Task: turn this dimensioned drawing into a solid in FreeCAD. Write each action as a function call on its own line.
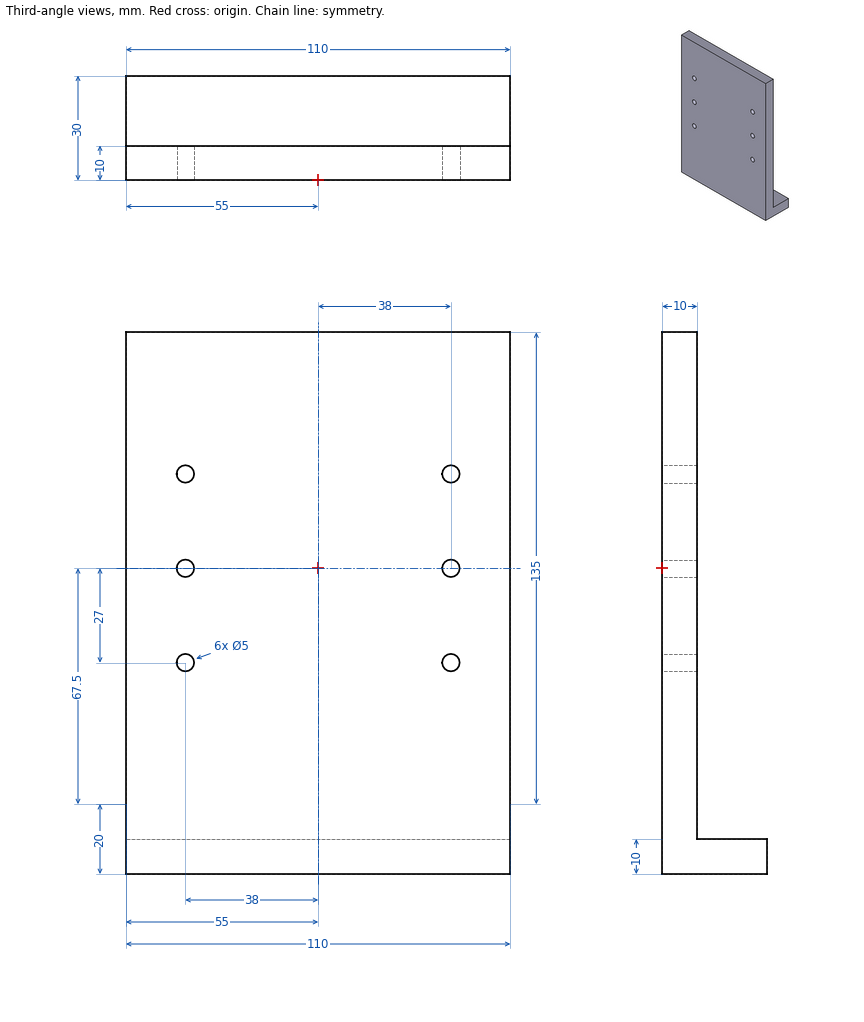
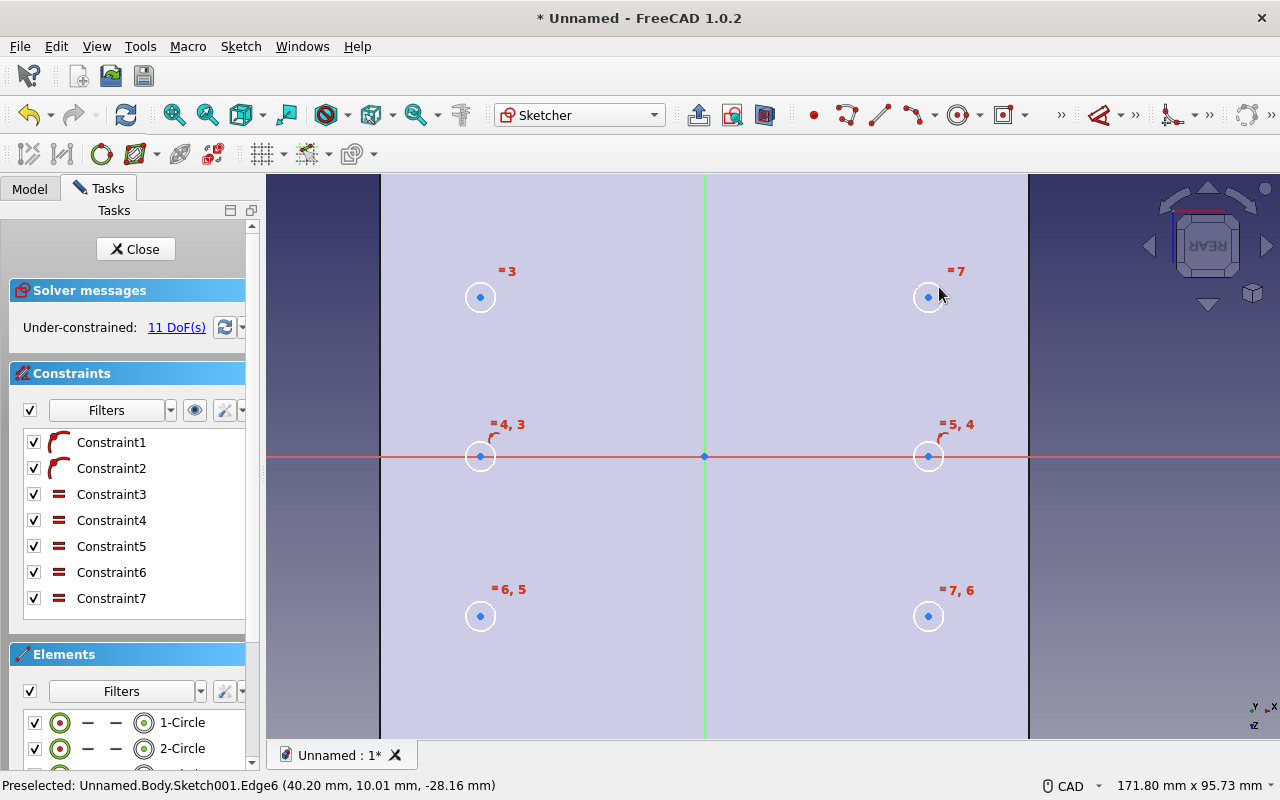
click(481, 298)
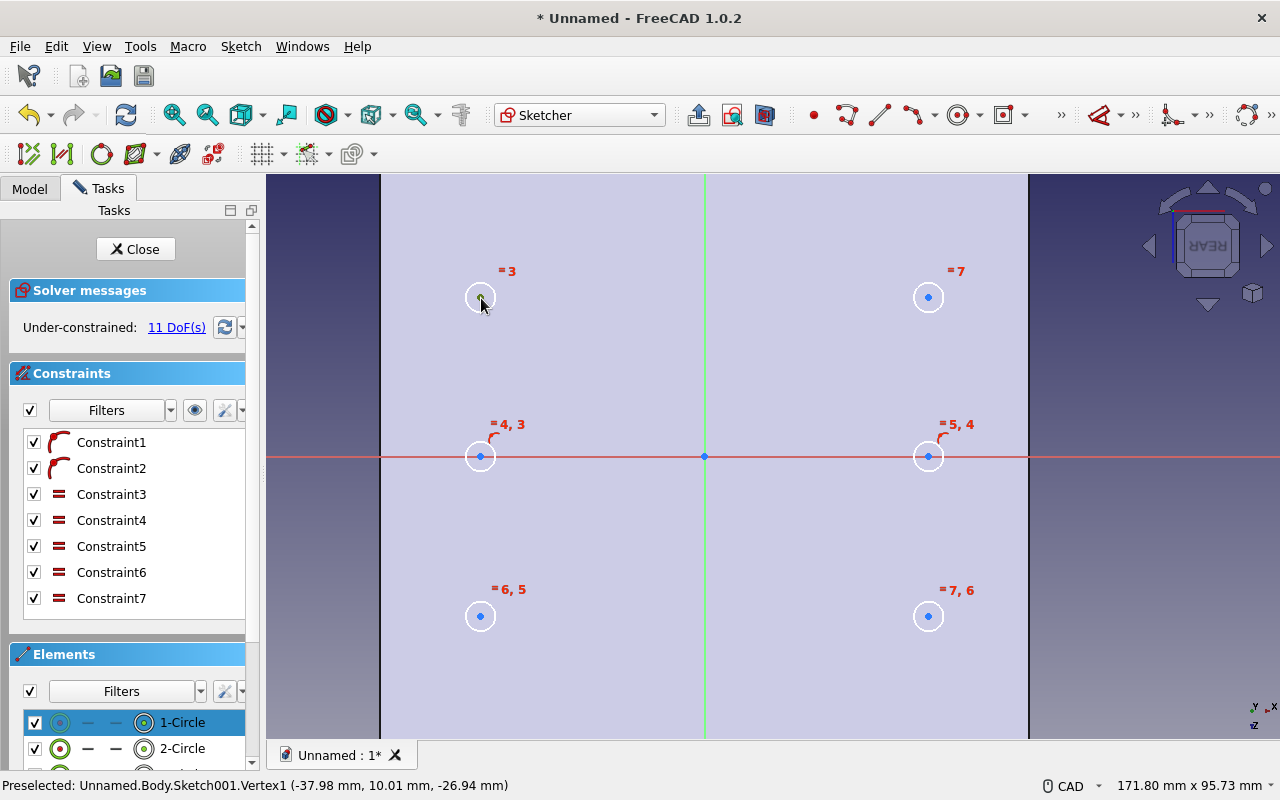
click(481, 616)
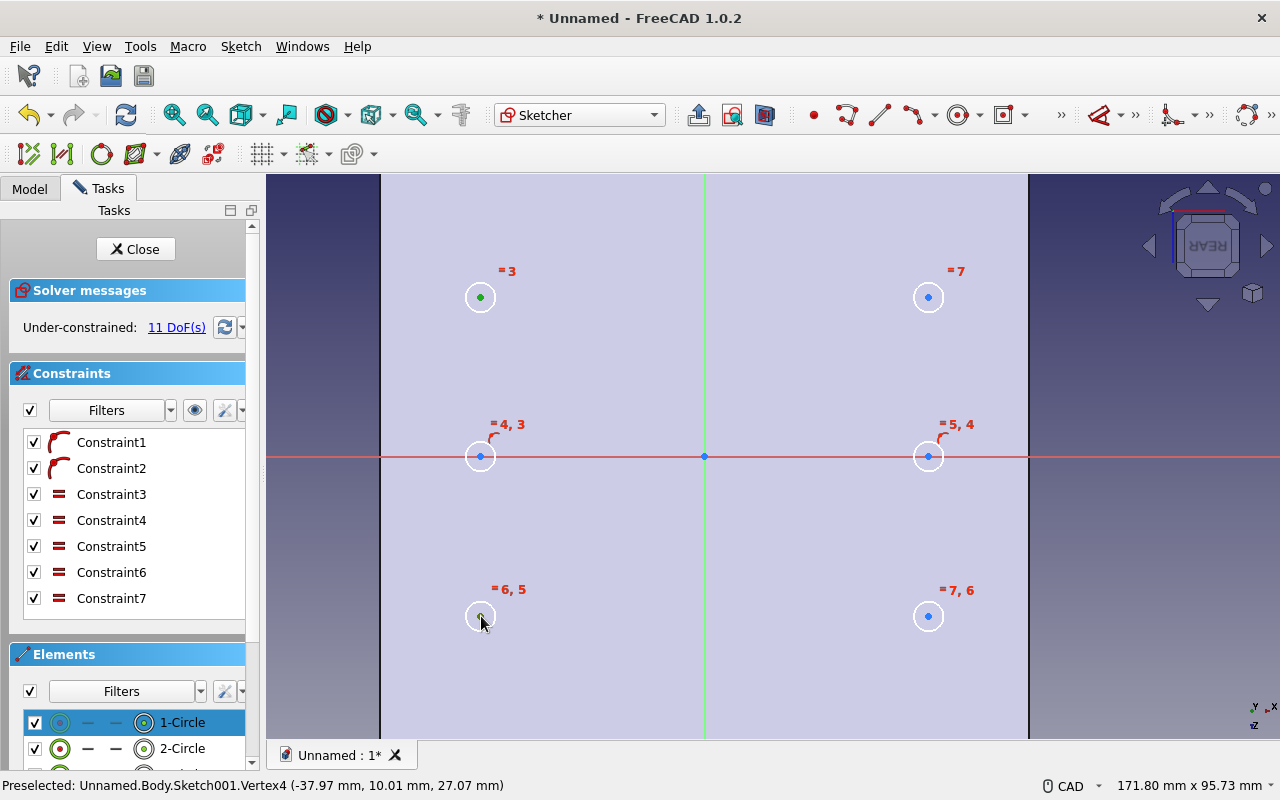
click(353, 457)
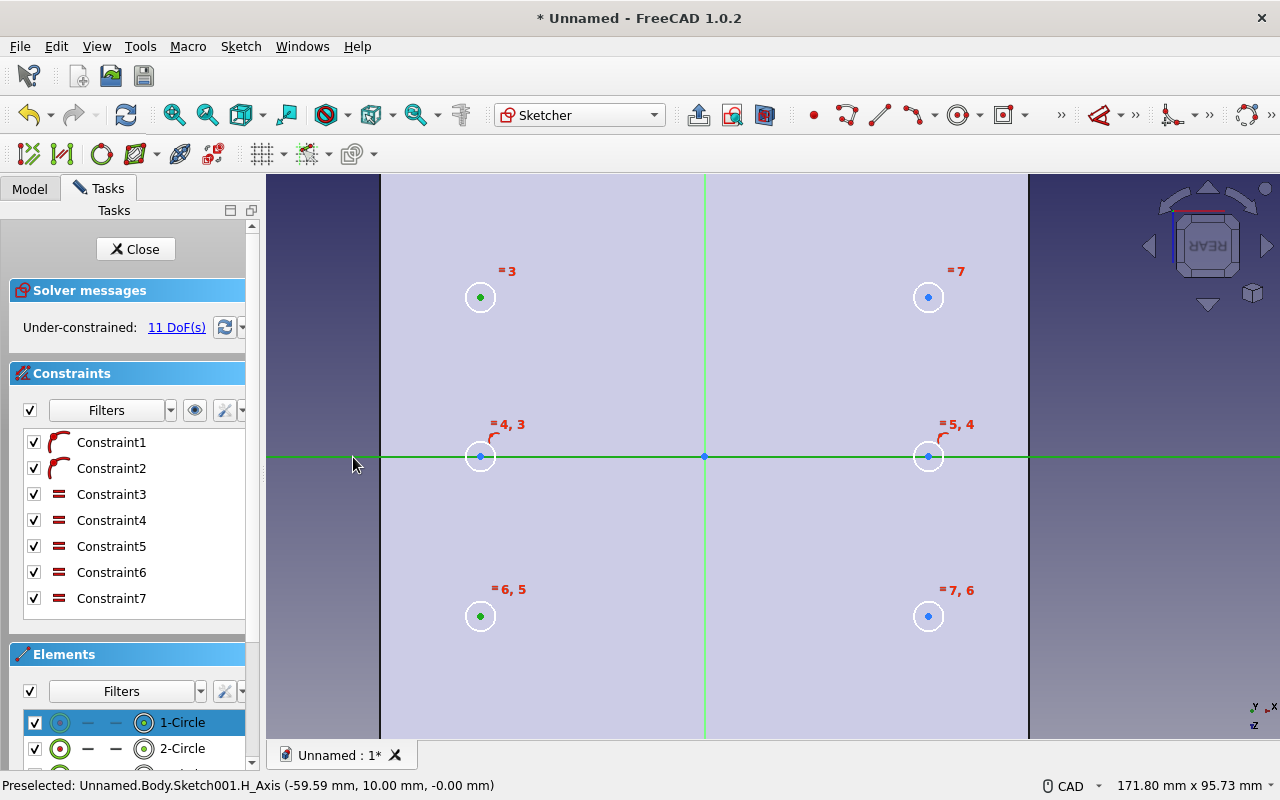
key(s)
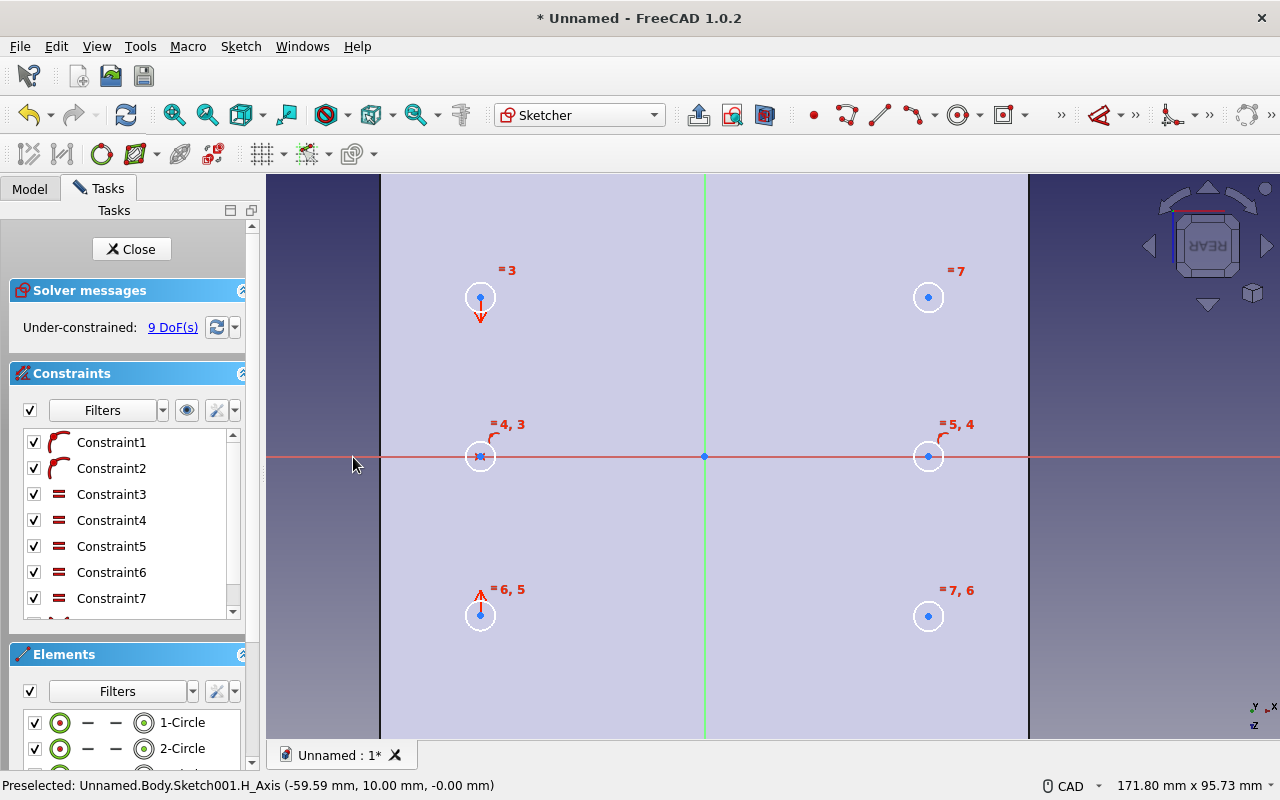
click(481, 616)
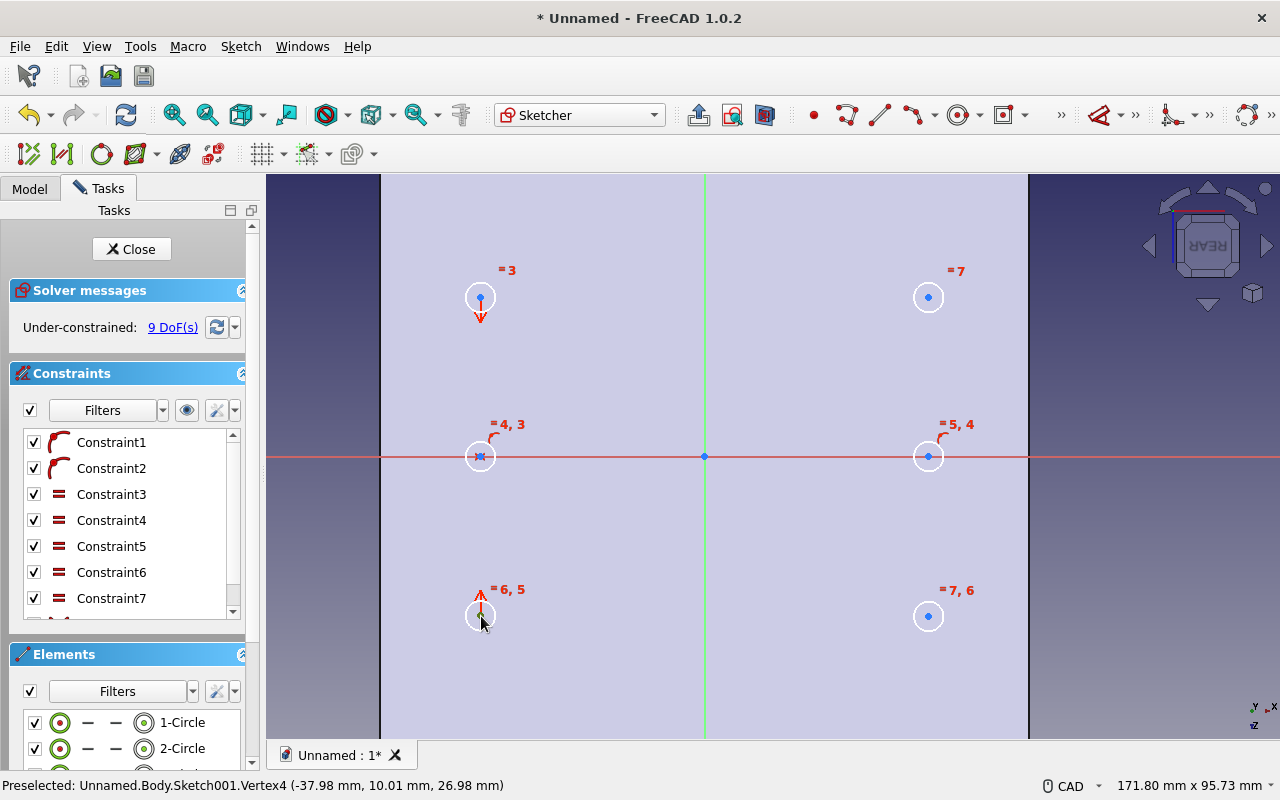
click(929, 616)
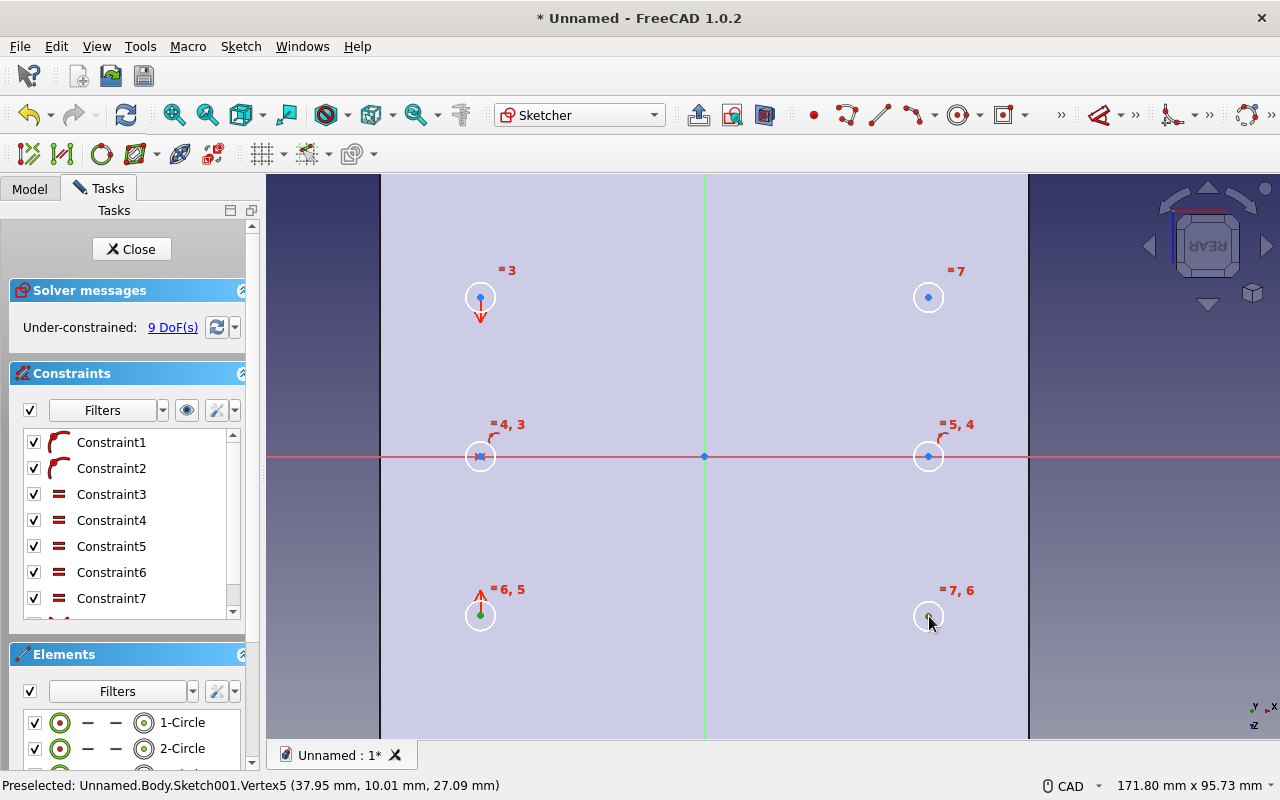
click(705, 675)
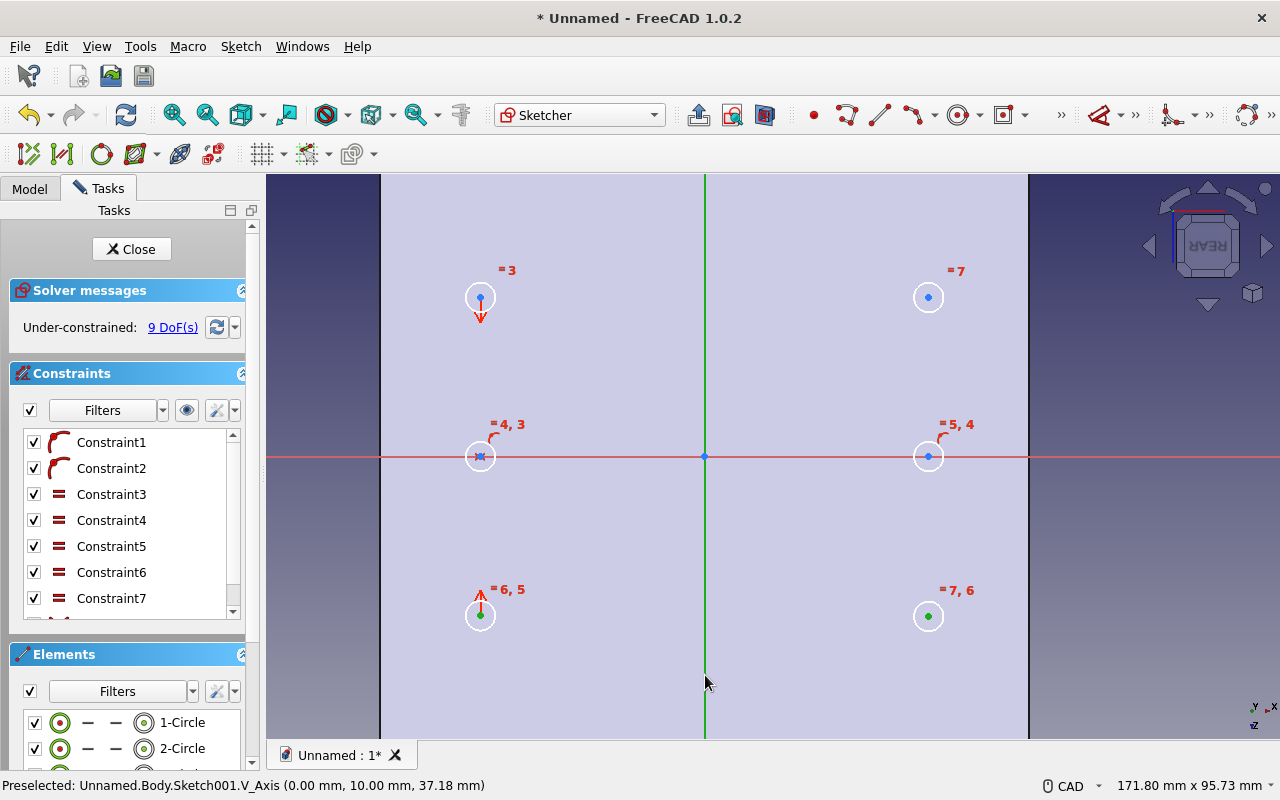
key(s)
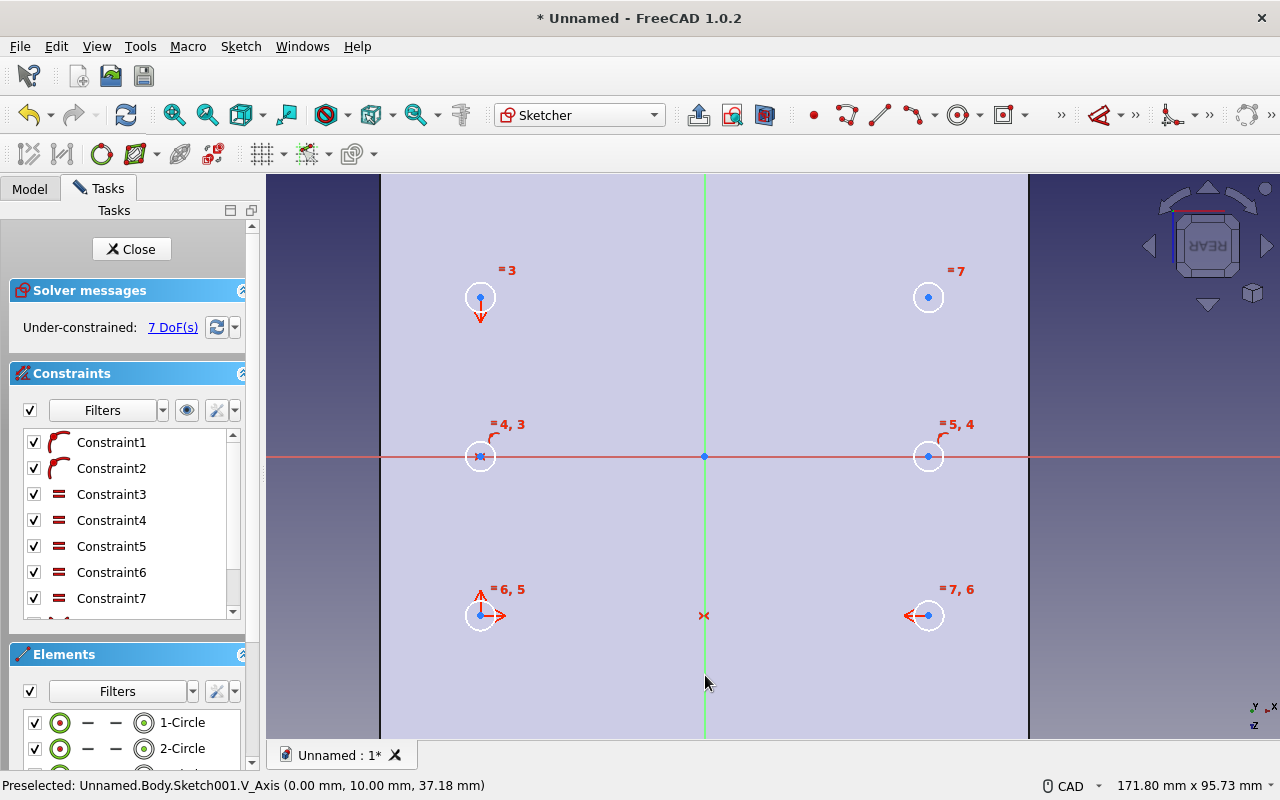
click(481, 297)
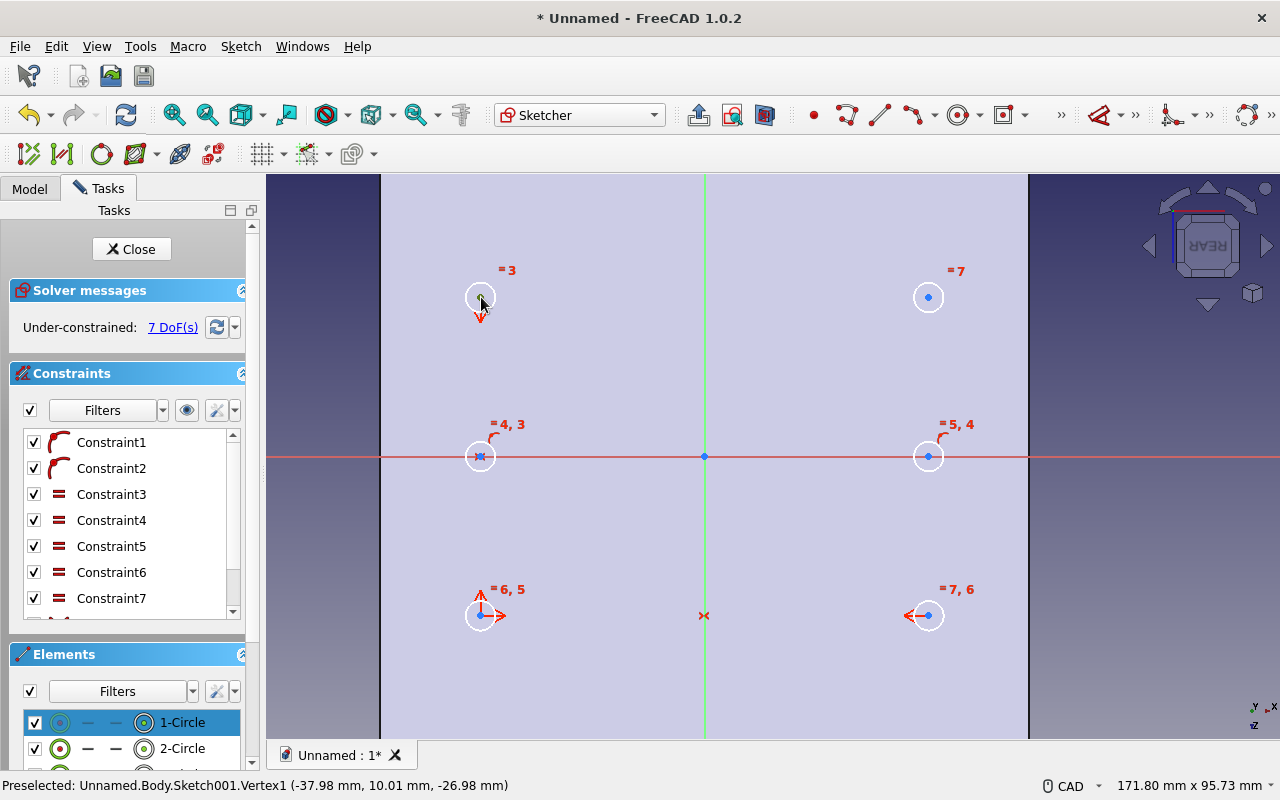
click(929, 298)